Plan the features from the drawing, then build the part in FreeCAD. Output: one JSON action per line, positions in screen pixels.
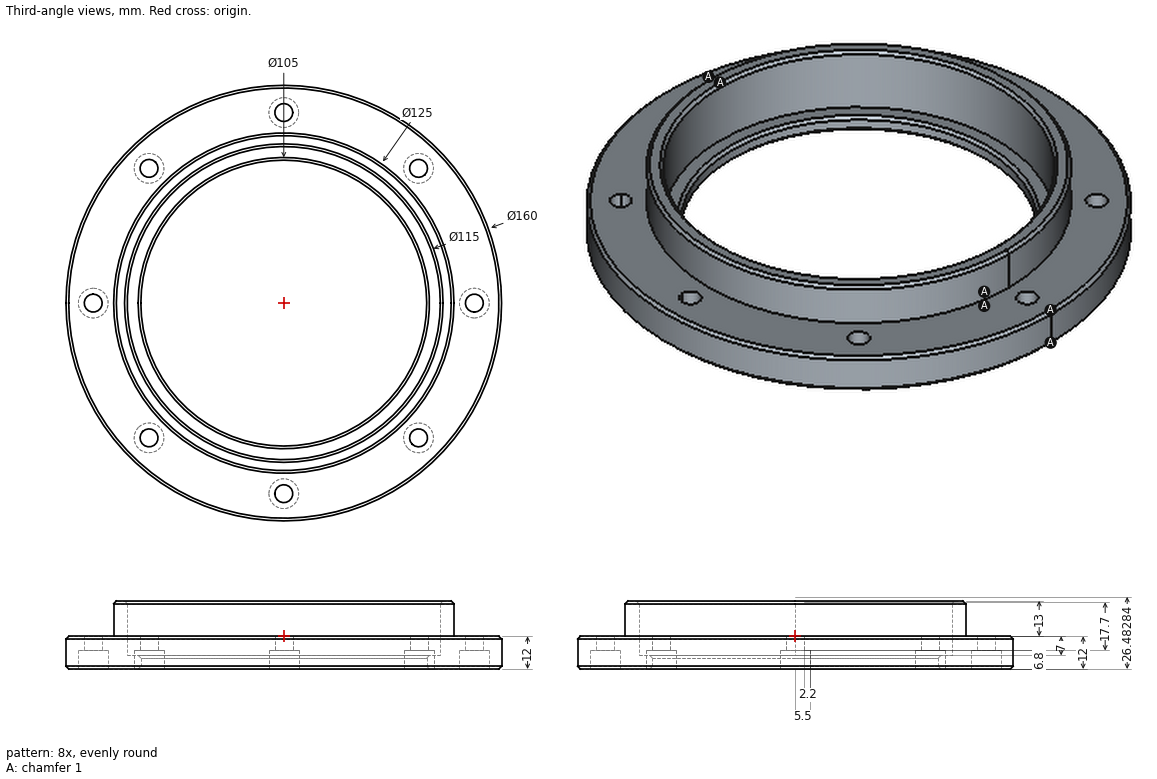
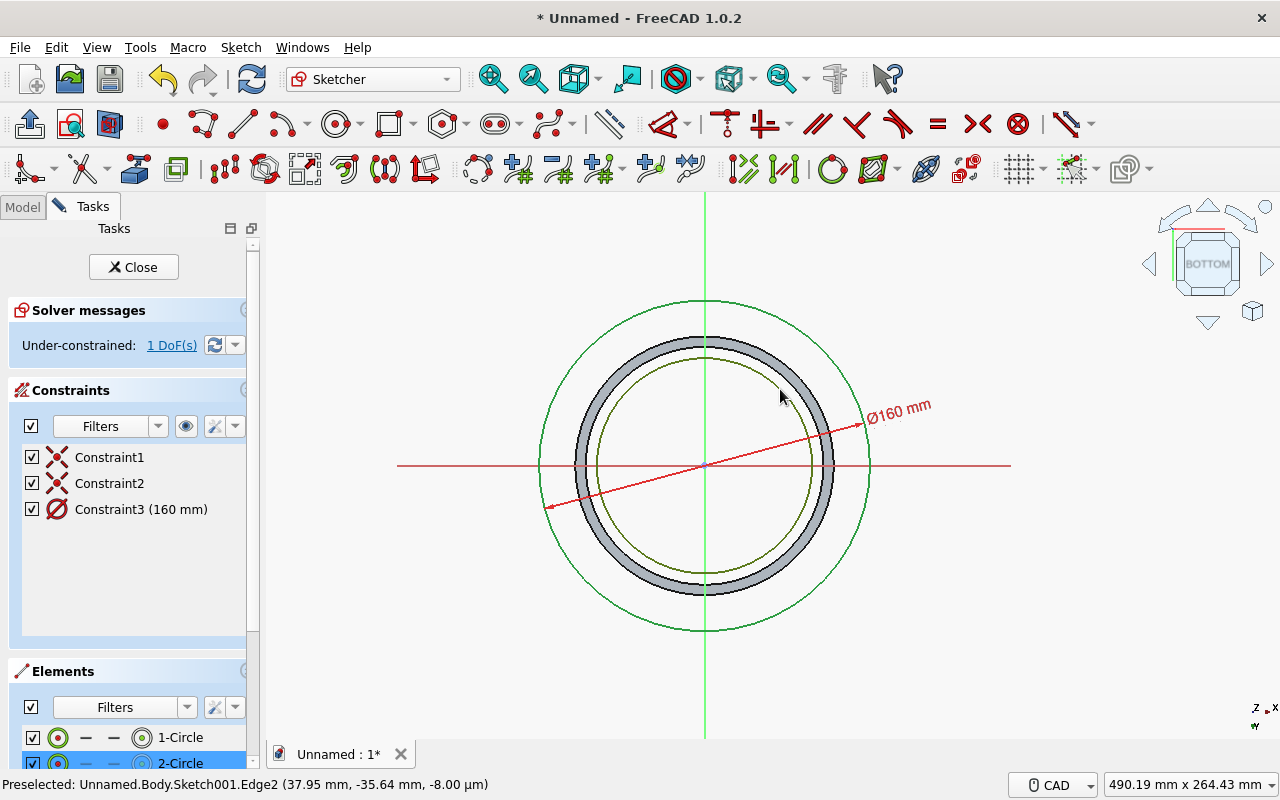
{"action": "key", "text": "k o"}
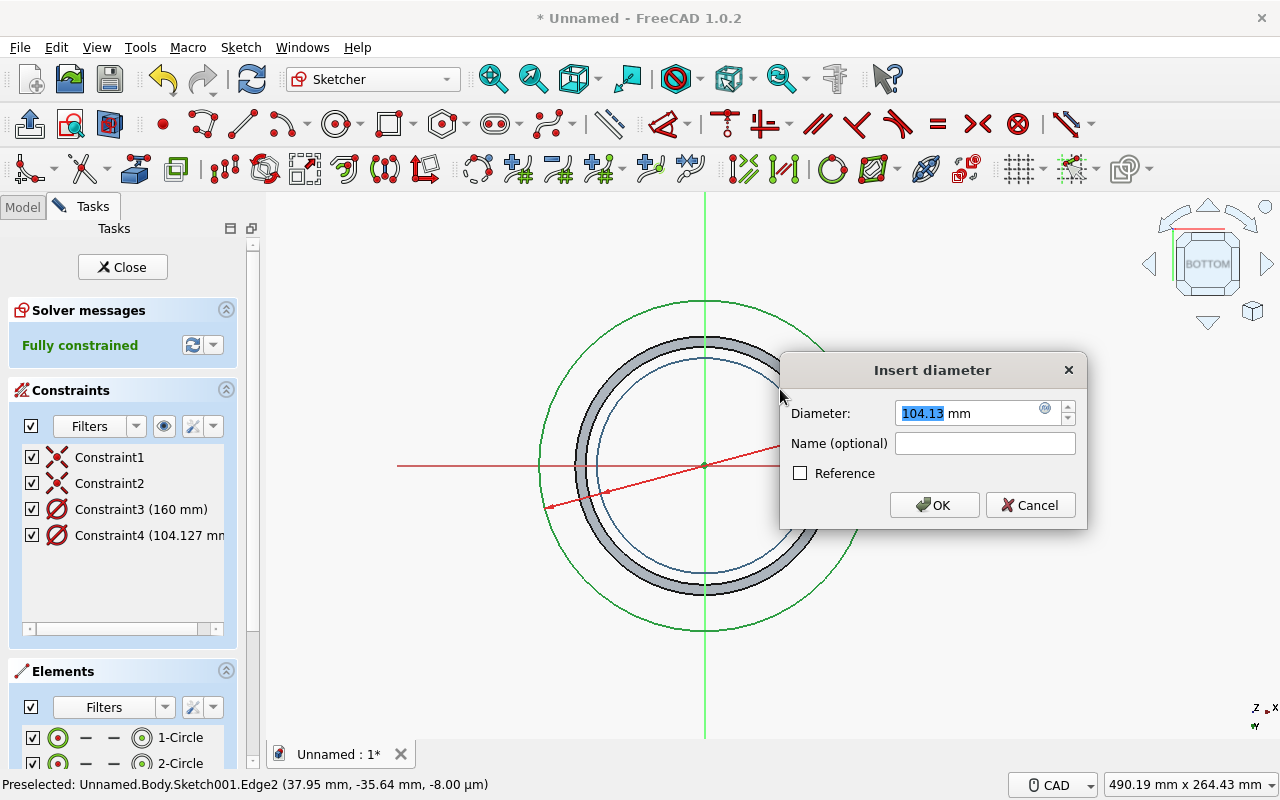
{"action": "type", "text": "105"}
{"action": "key", "text": "Return"}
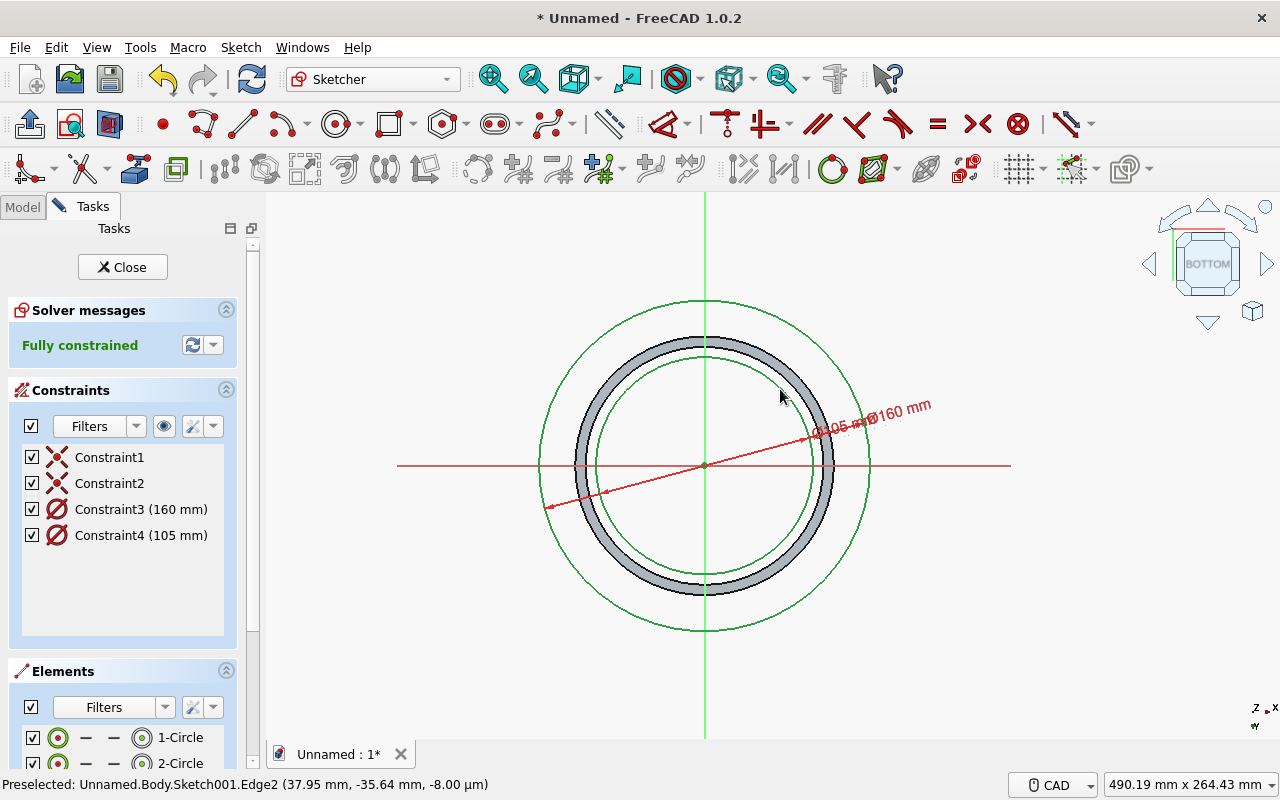
{"action": "left_click", "coordinate": [123, 267]}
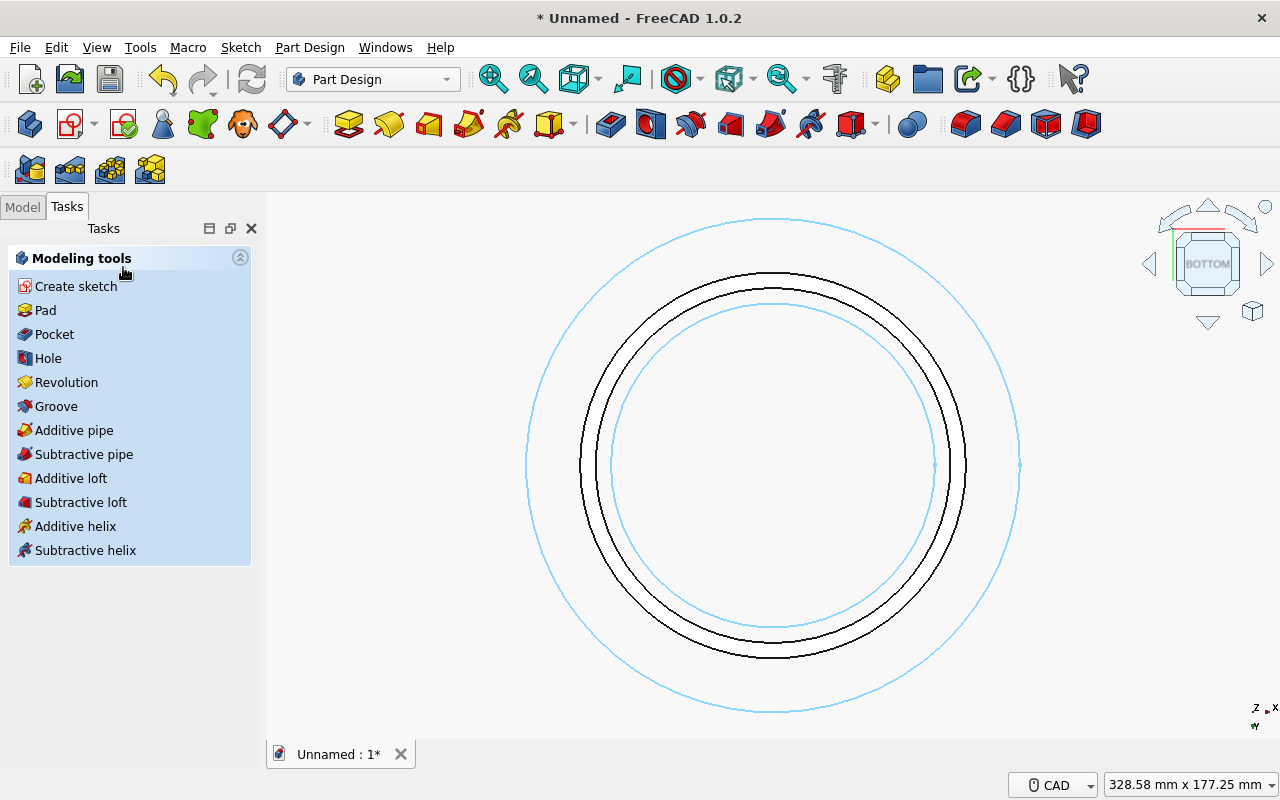
{"action": "left_click", "coordinate": [350, 124]}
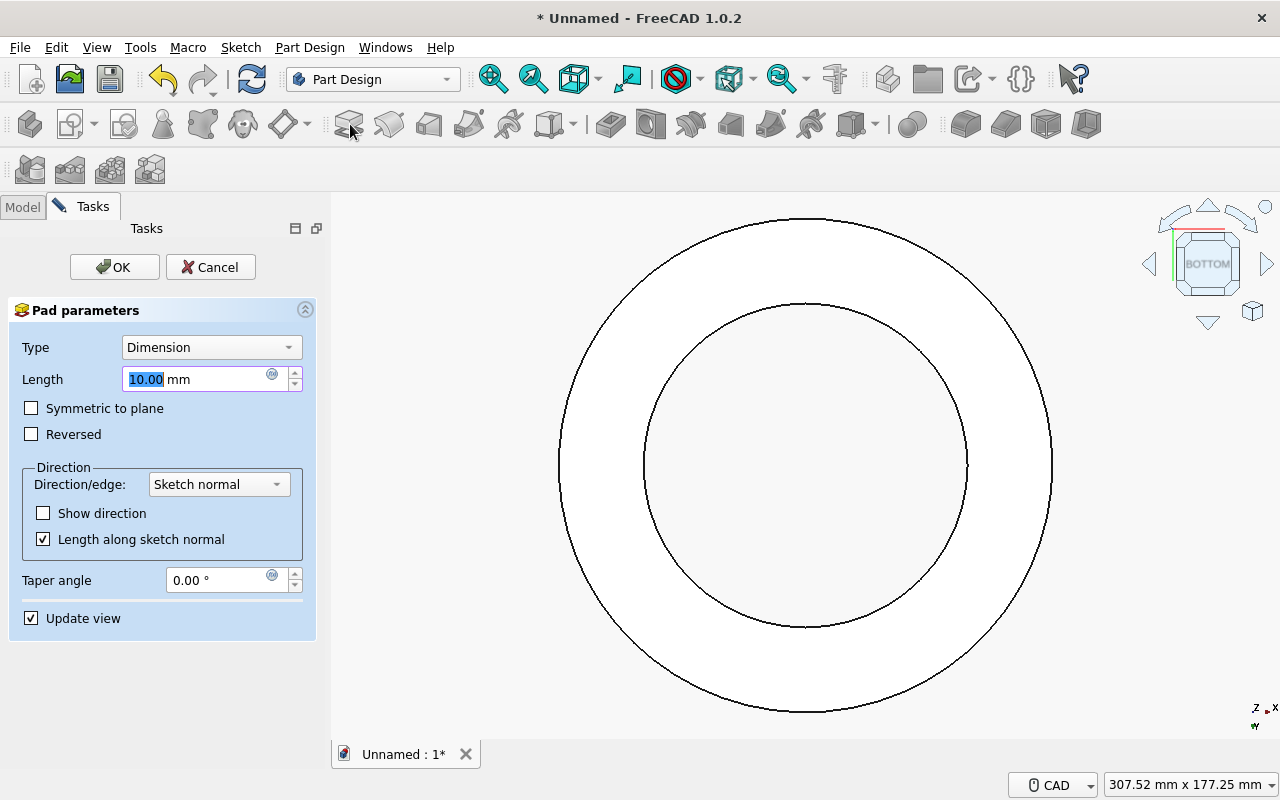
{"action": "type", "text": "12"}
{"action": "key", "text": "Tab"}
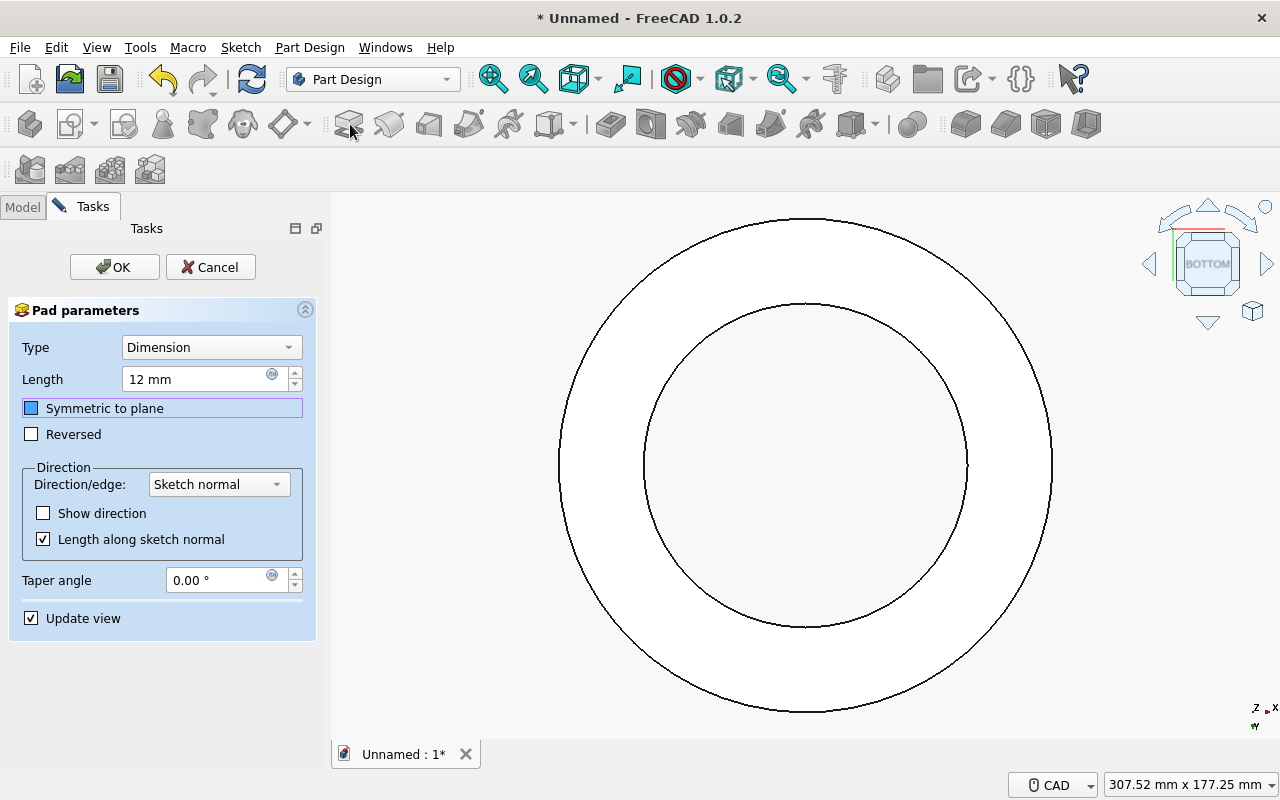
{"action": "left_click", "coordinate": [115, 267]}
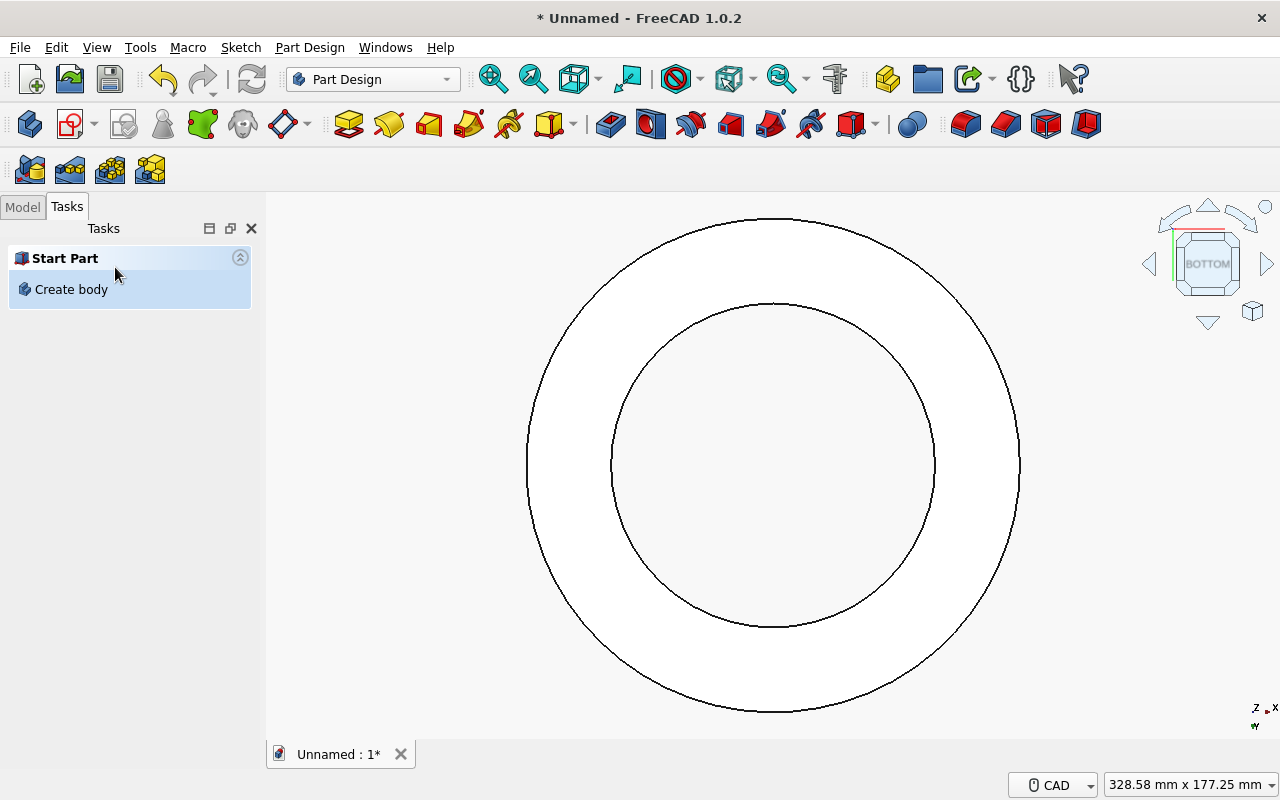
{"action": "left_click", "coordinate": [23, 206]}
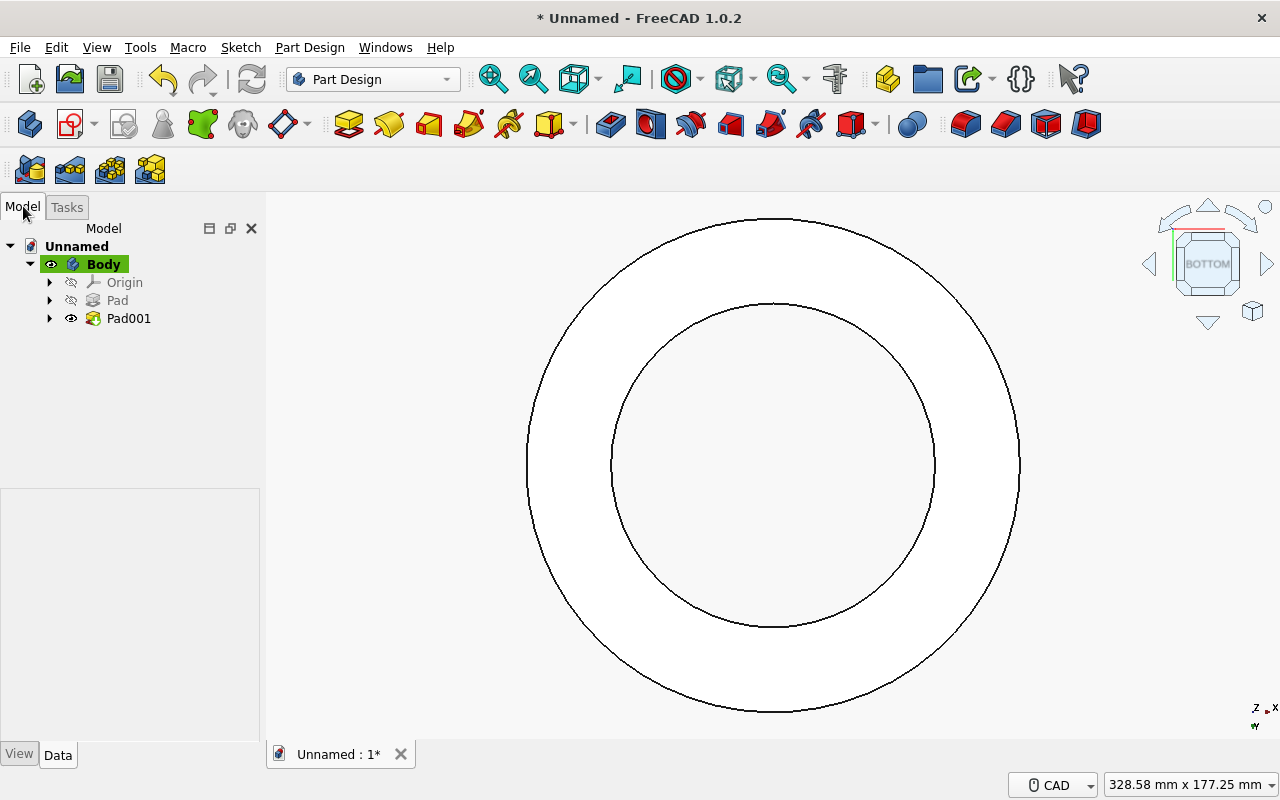
{"action": "left_click", "coordinate": [50, 282]}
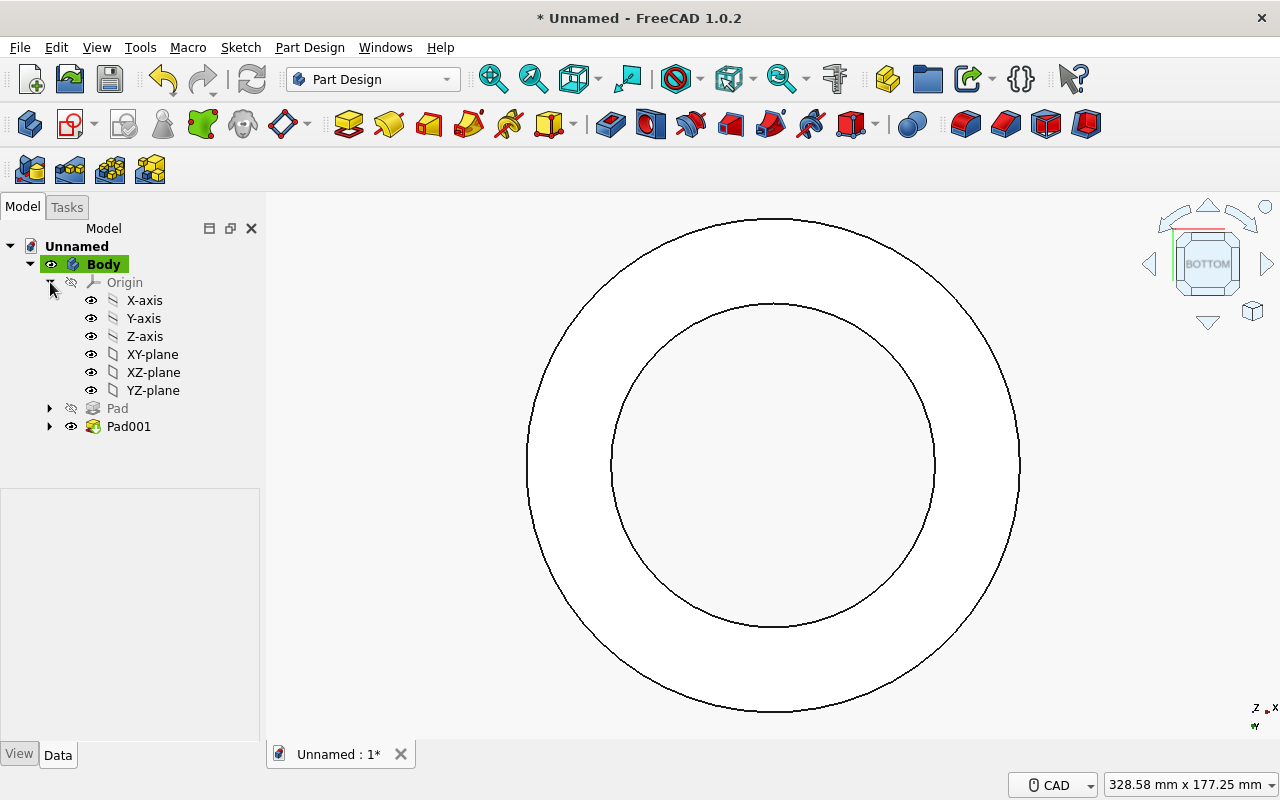
{"action": "left_click", "coordinate": [136, 354]}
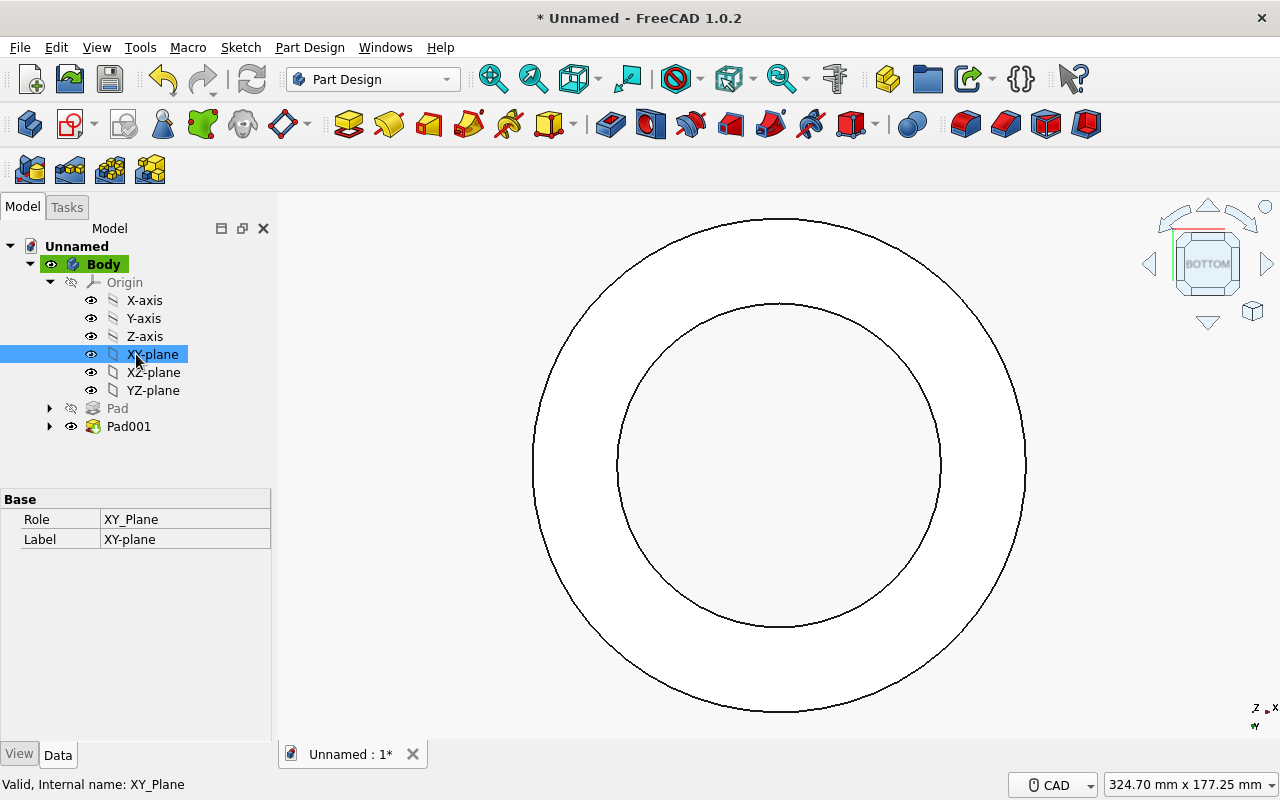
{"action": "left_click", "coordinate": [284, 124]}